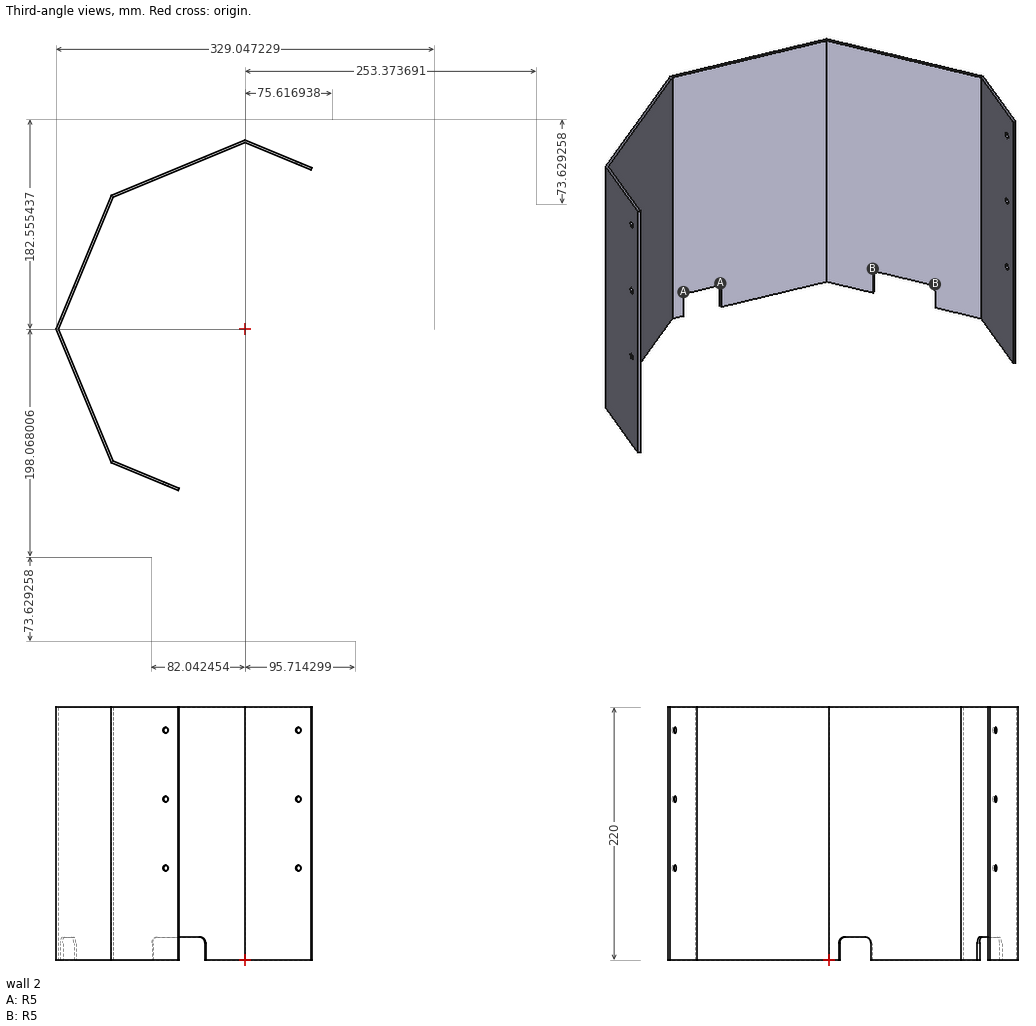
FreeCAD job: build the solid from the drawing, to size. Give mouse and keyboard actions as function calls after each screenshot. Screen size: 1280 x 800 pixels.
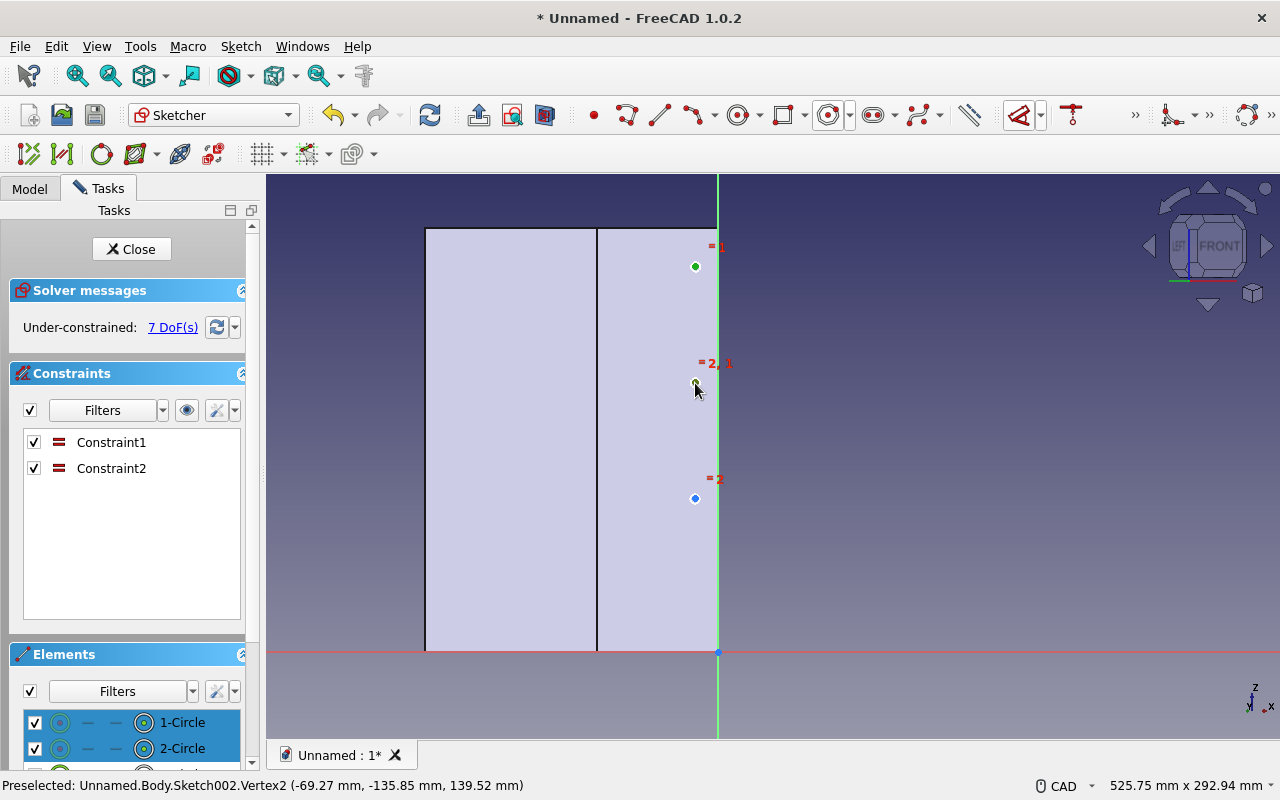
key(v)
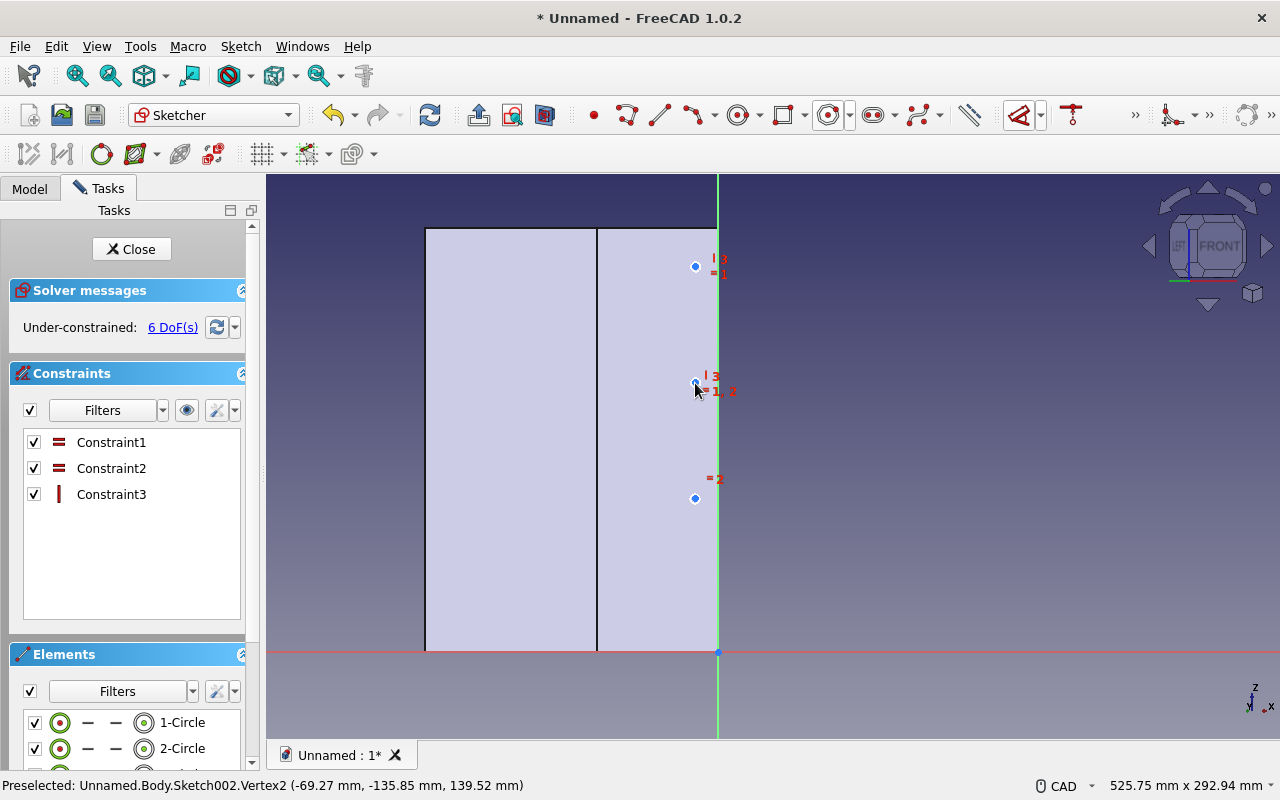
click(696, 383)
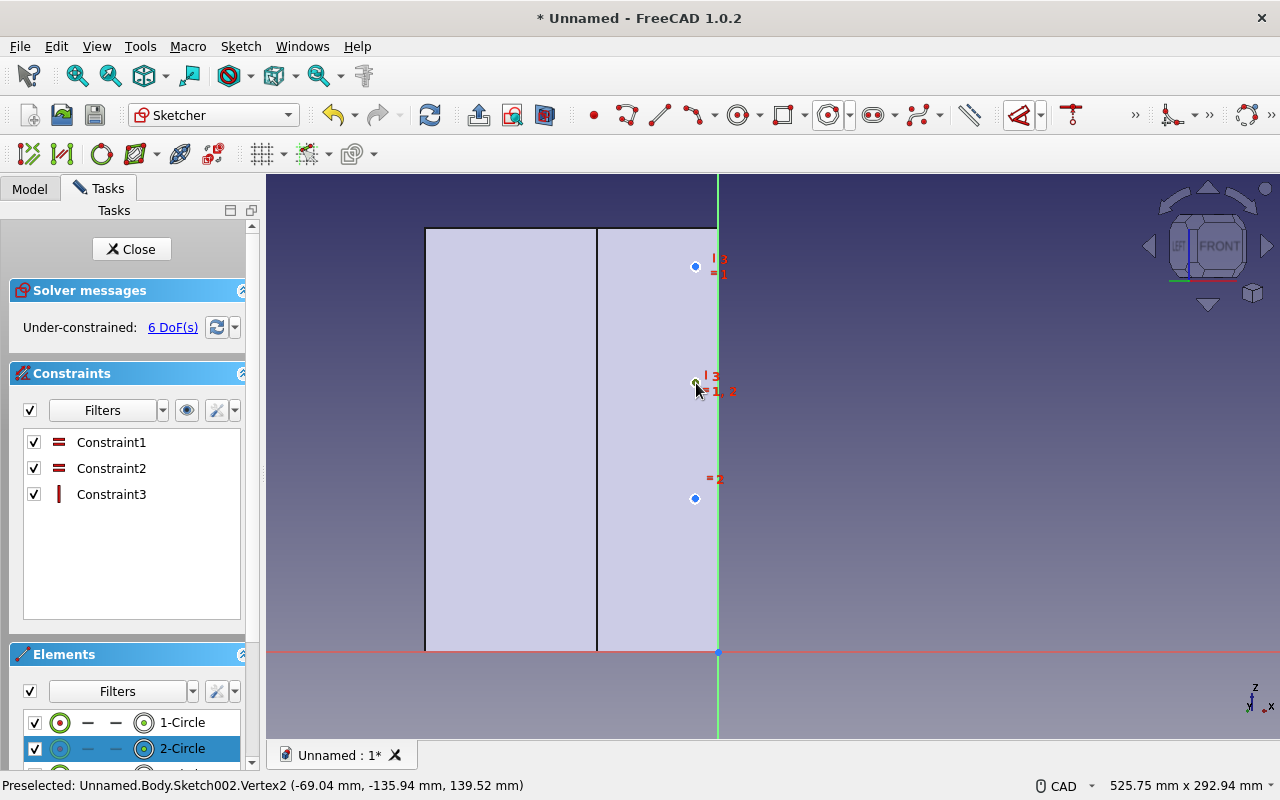
click(695, 499)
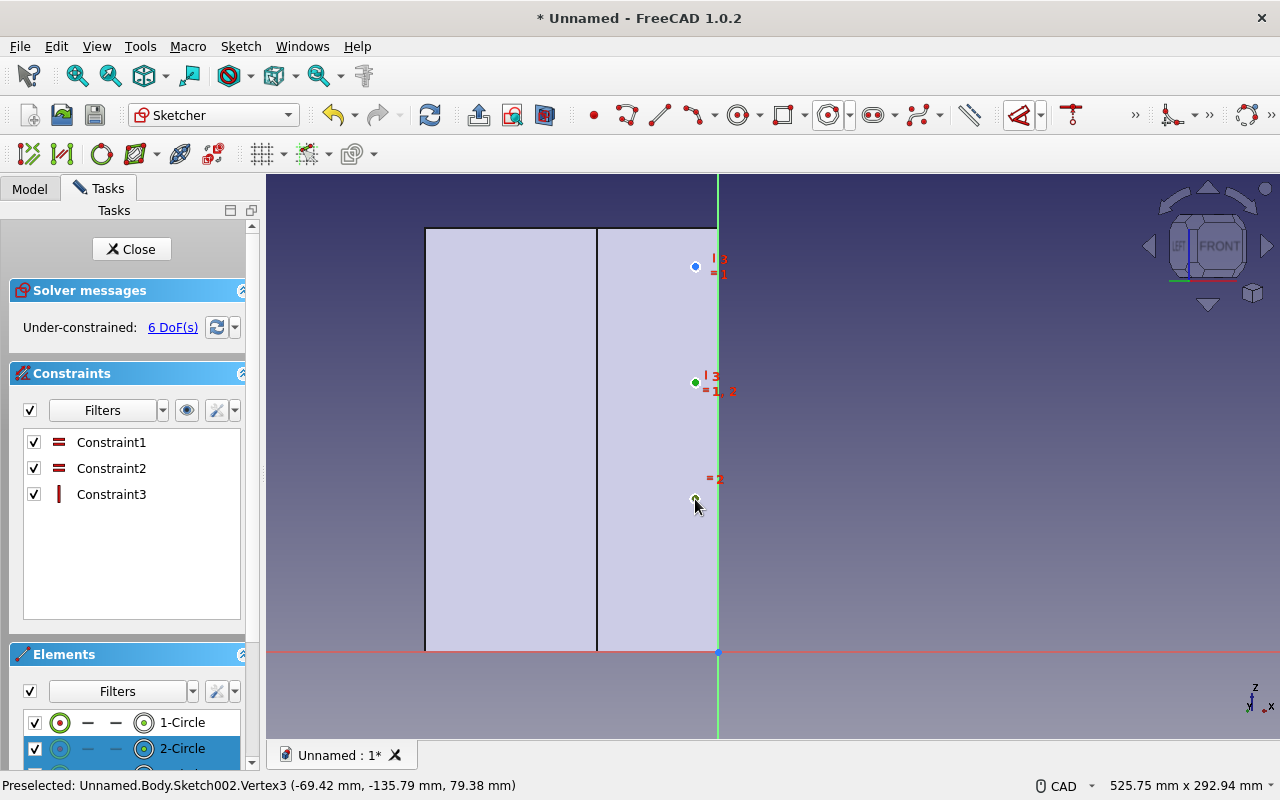
key(v)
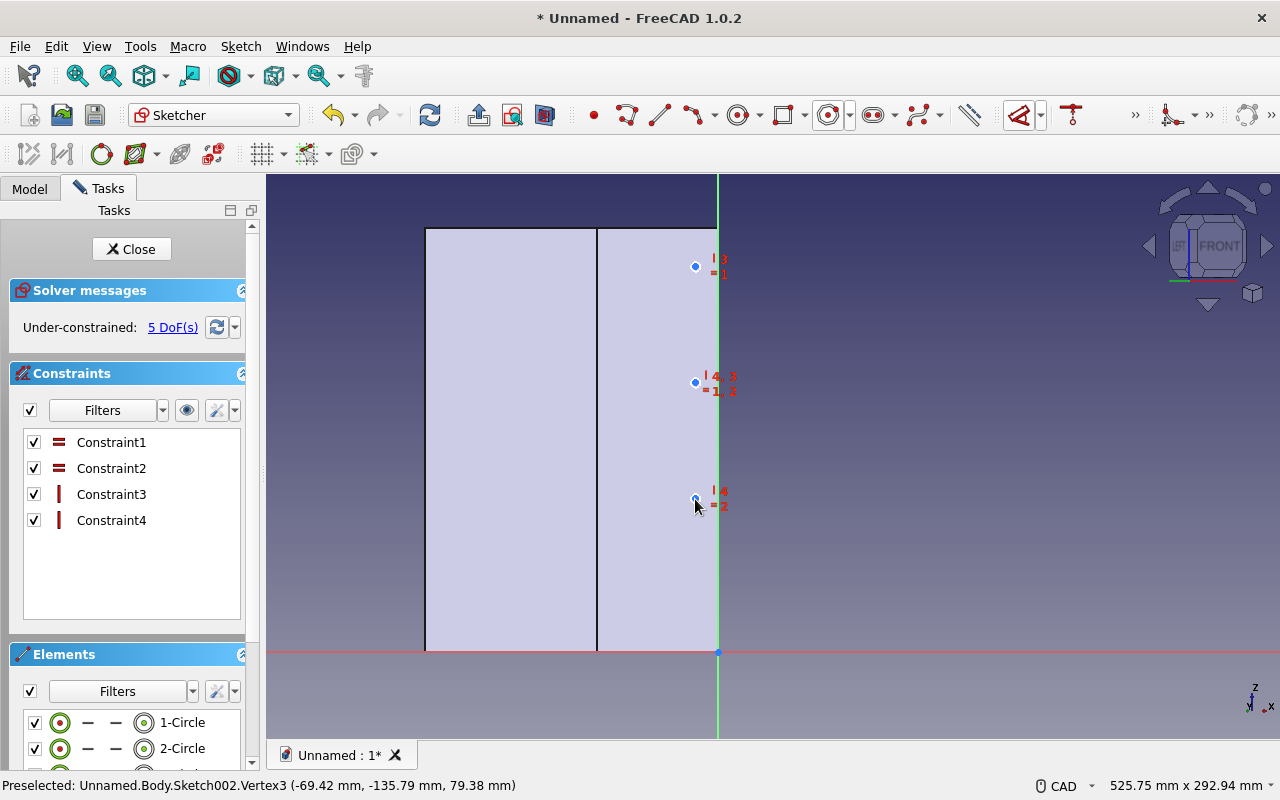
scroll(692, 264, up, 8)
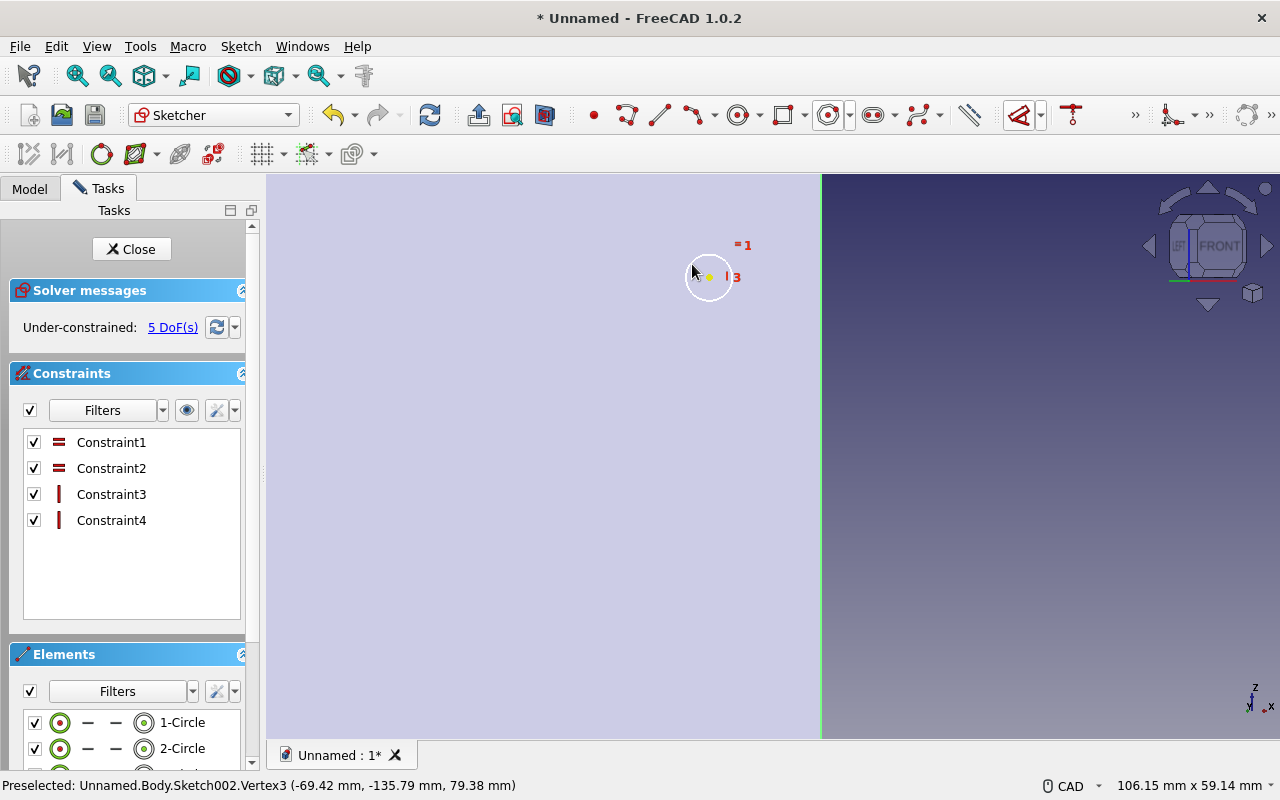
click(693, 261)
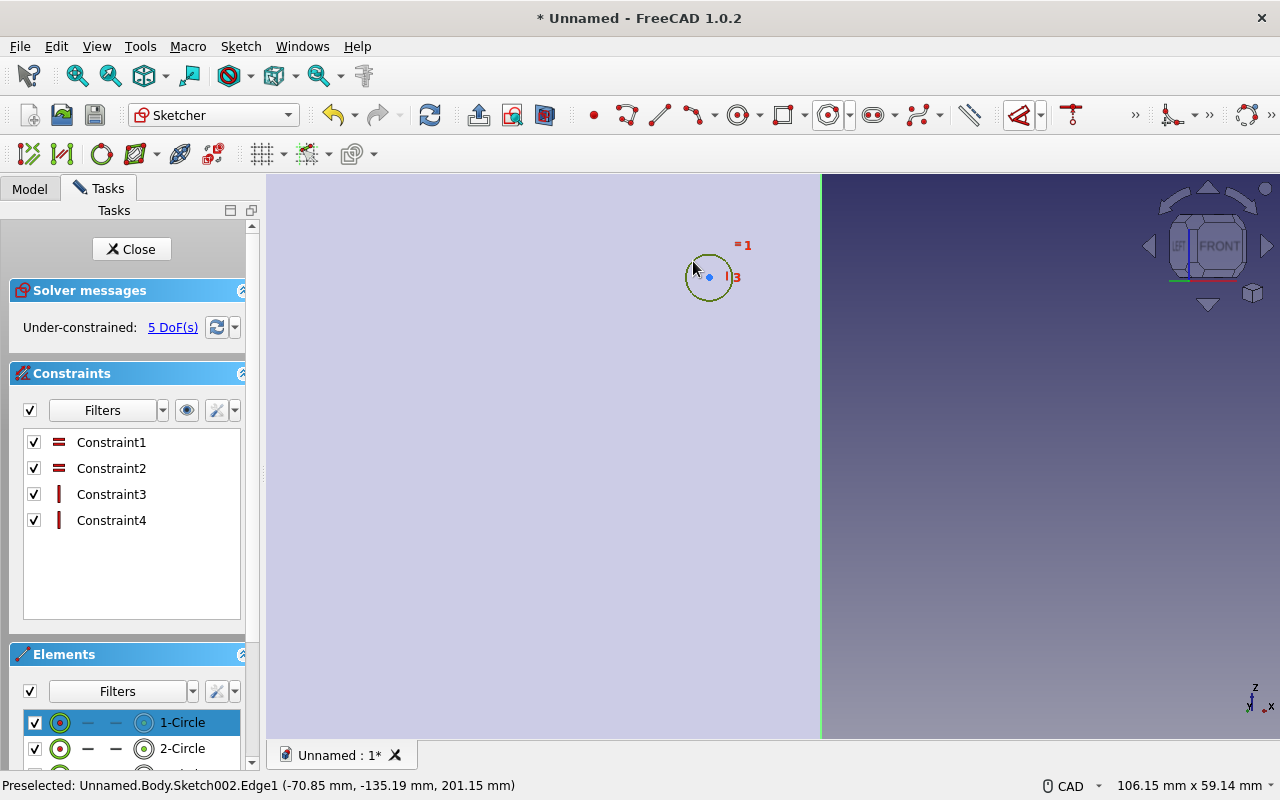
key(k)
key(o)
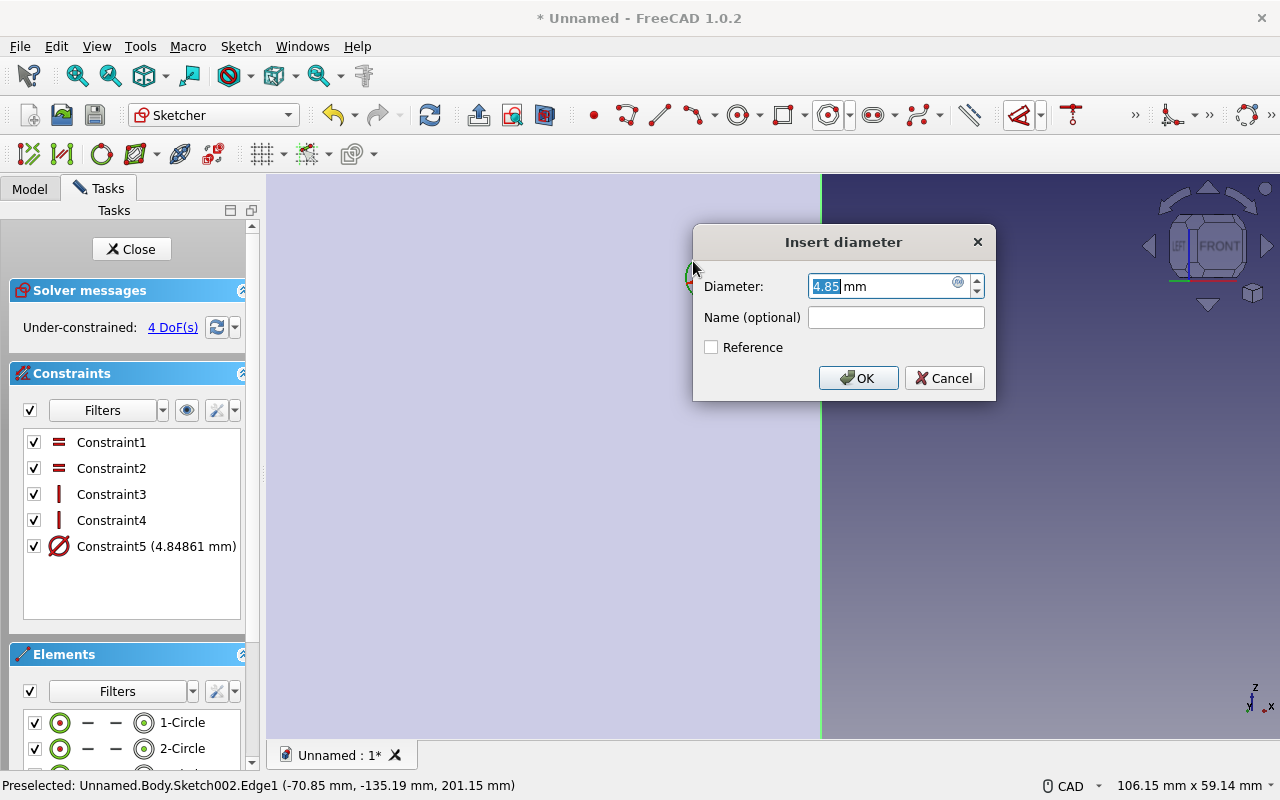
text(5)
key(Return)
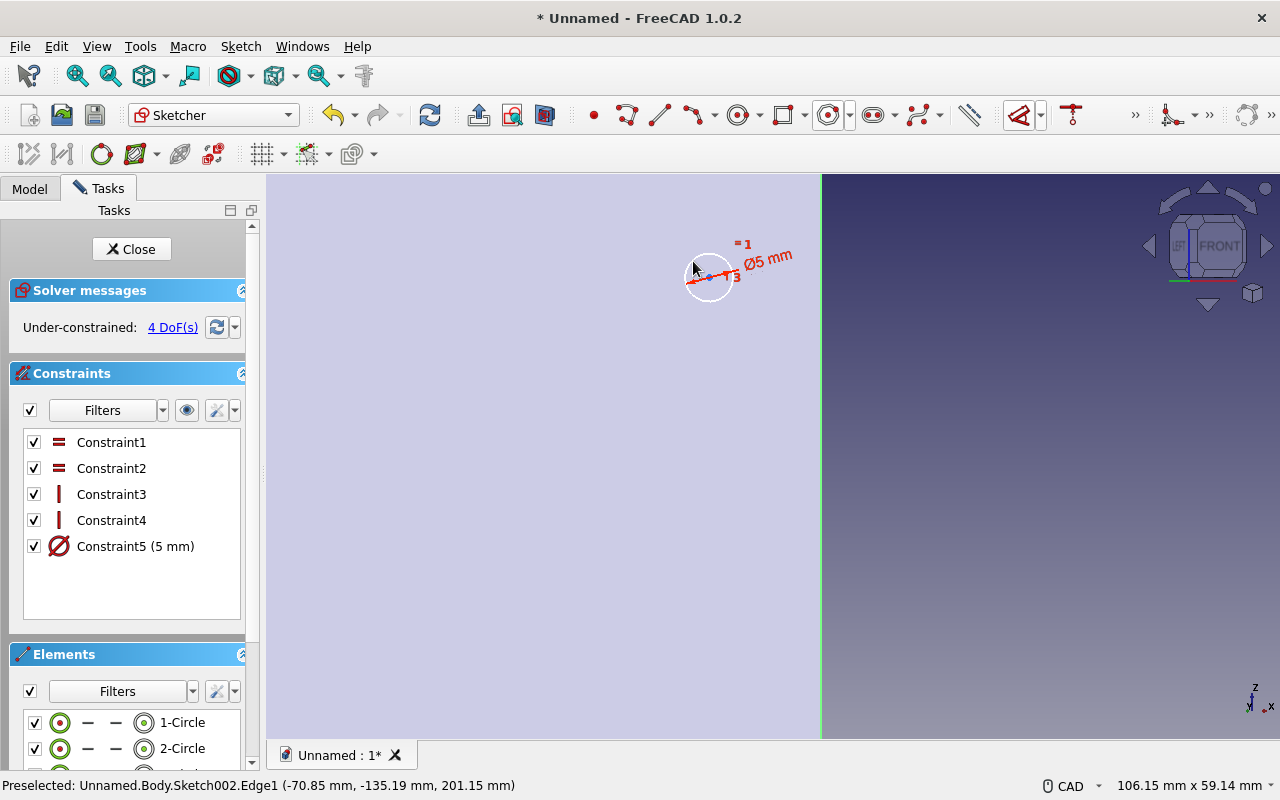
scroll(692, 264, down, 8)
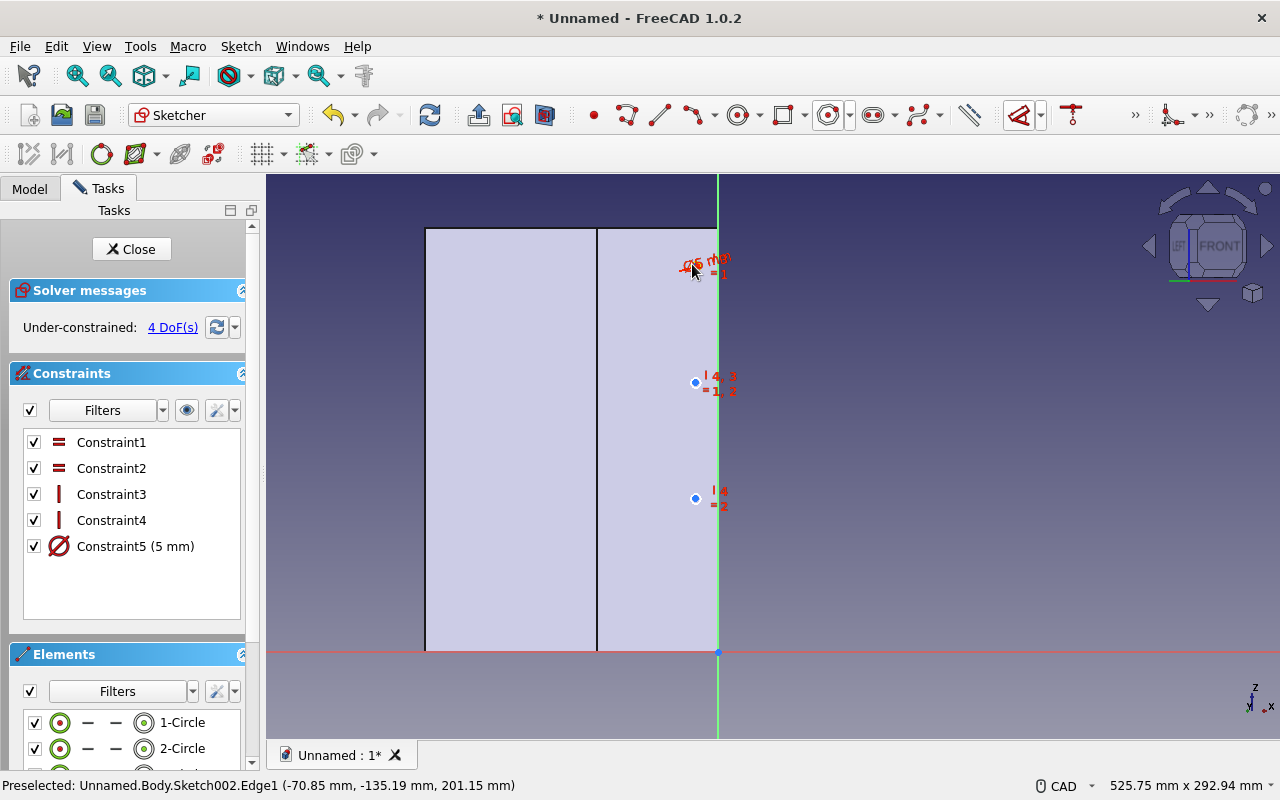
scroll(696, 267, up, 3)